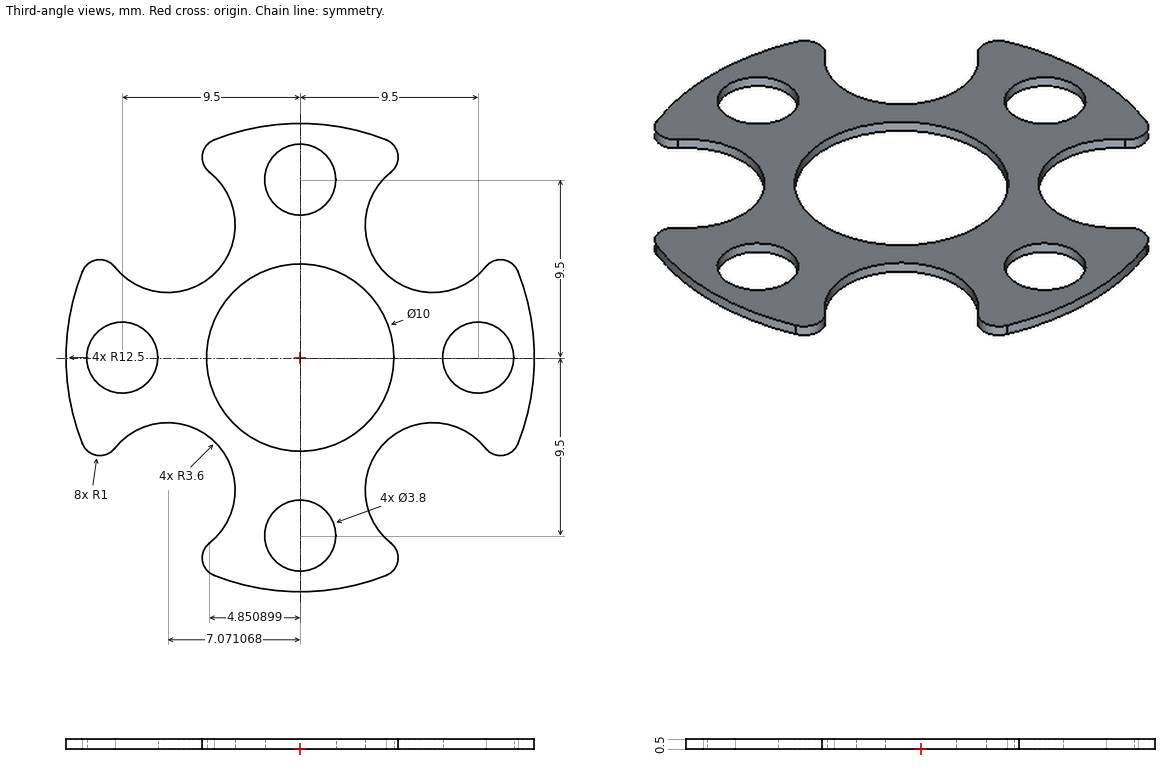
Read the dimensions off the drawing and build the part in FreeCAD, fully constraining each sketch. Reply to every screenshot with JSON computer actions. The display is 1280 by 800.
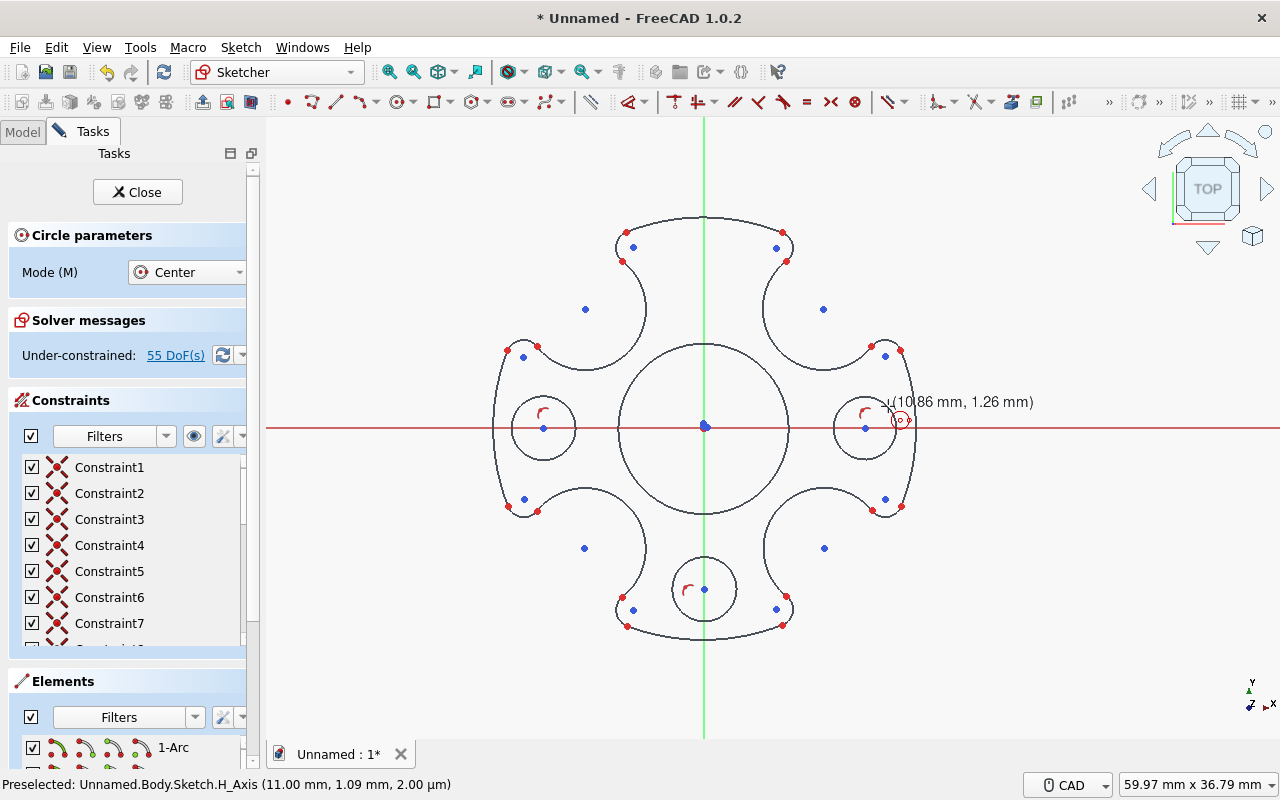
{"action": "left_click", "coordinate": [704, 268]}
{"action": "left_click", "coordinate": [727, 245]}
{"action": "key", "text": "Escape"}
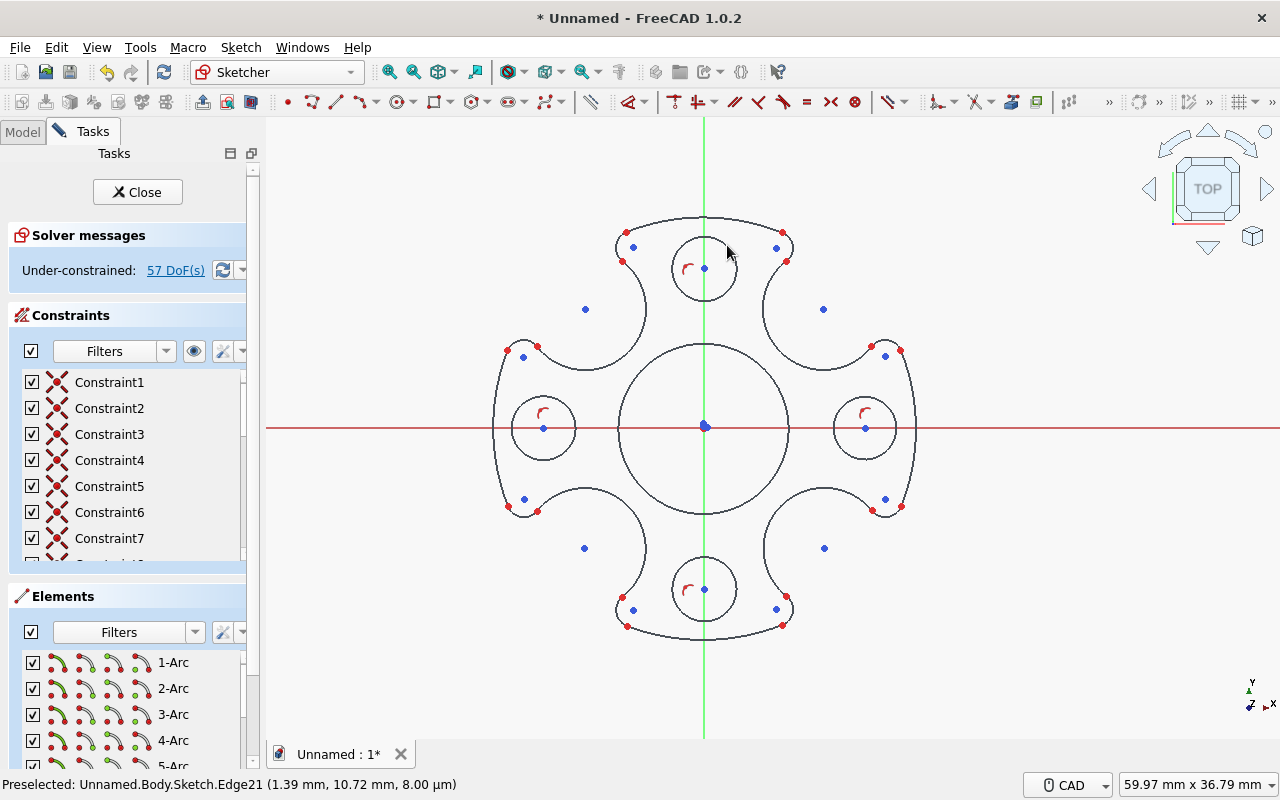
{"action": "left_click", "coordinate": [645, 543]}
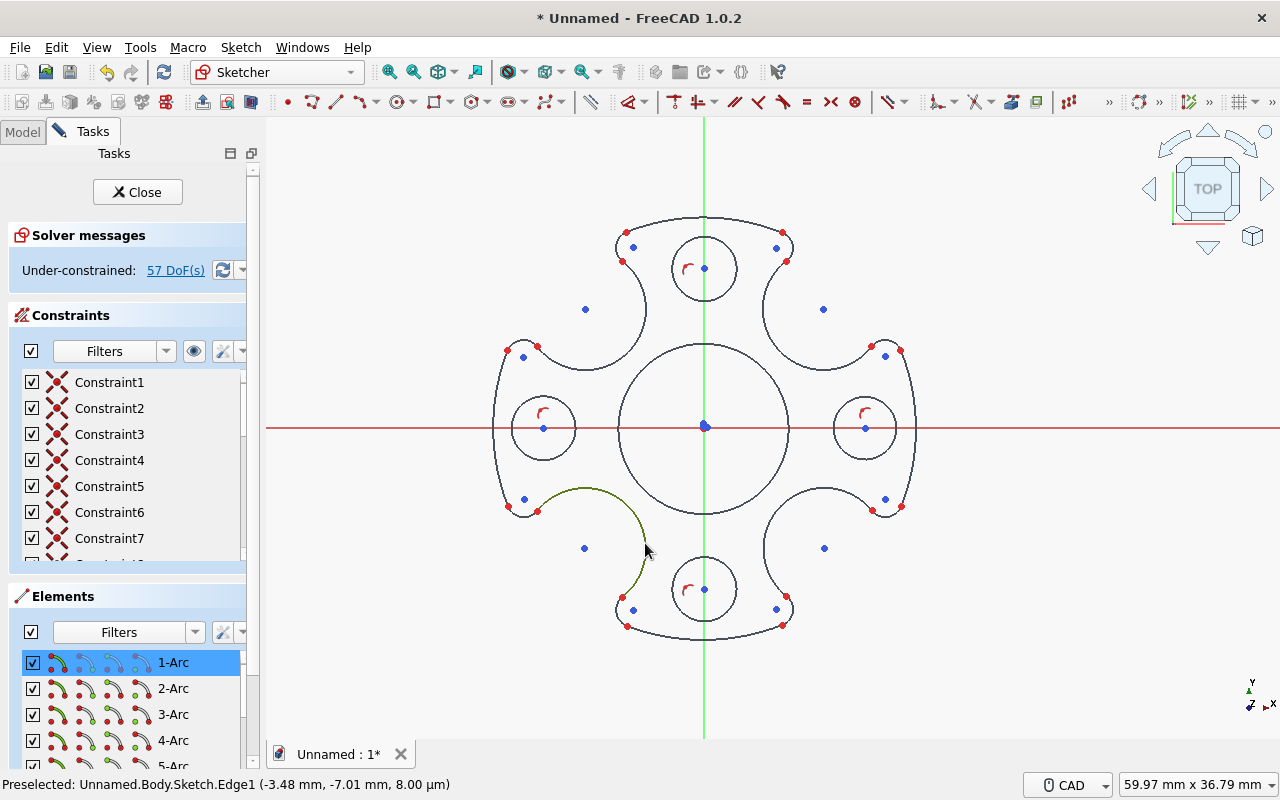
{"action": "scroll", "coordinate": [617, 606], "scroll_direction": "up", "scroll_amount": 2}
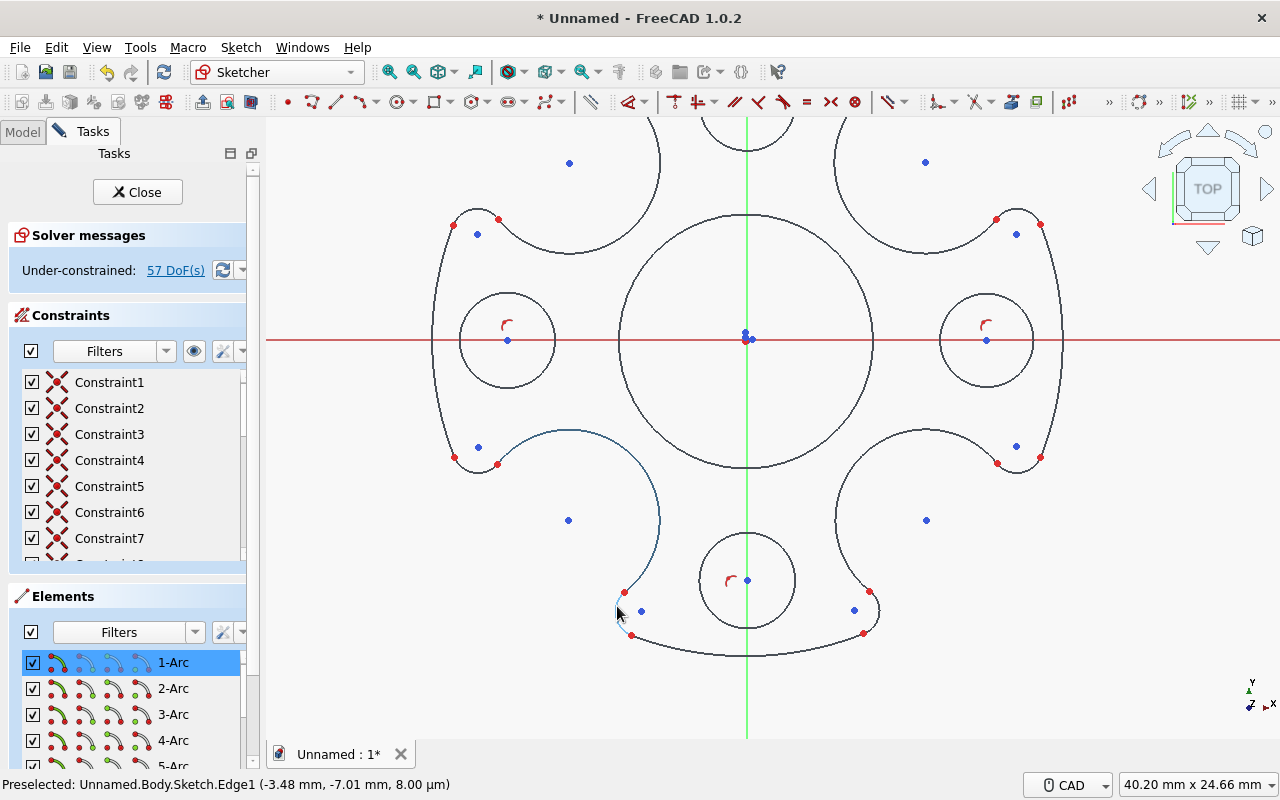
{"action": "left_click", "coordinate": [616, 606]}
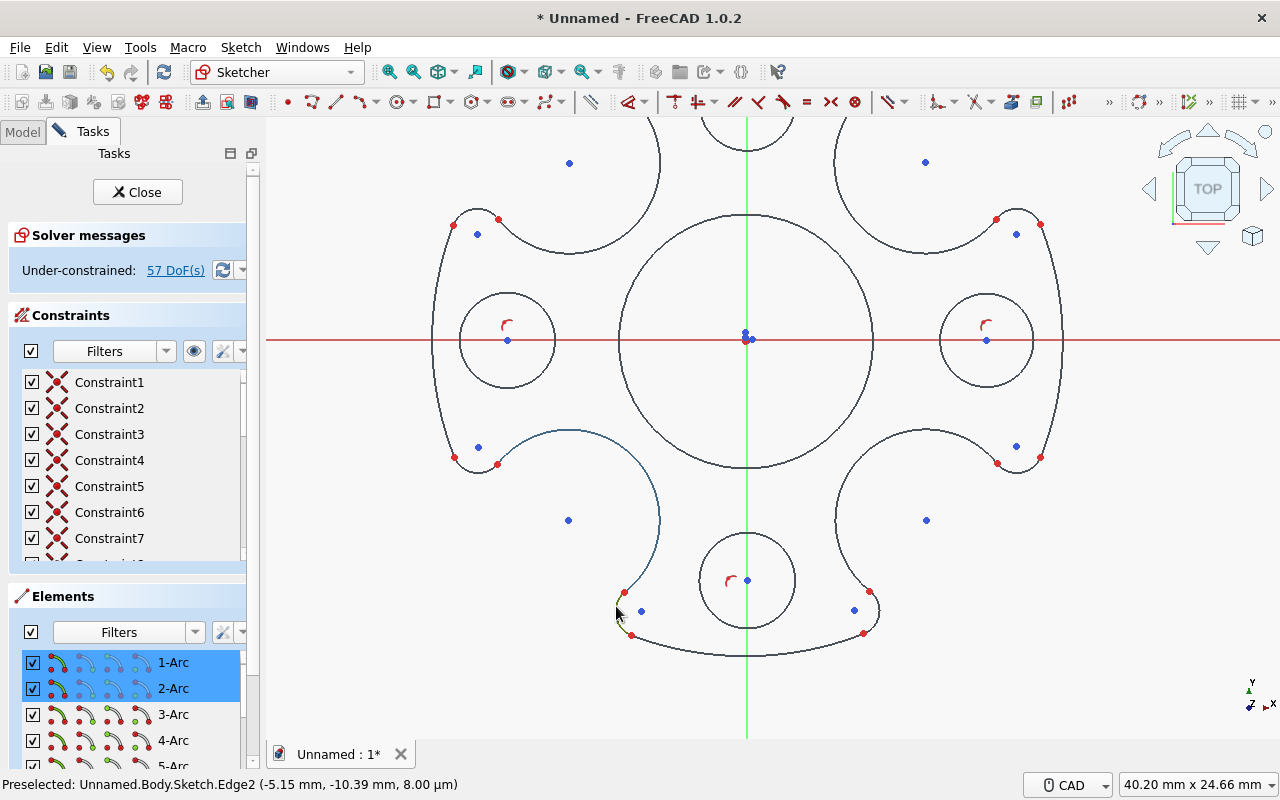
{"action": "left_click", "coordinate": [784, 102]}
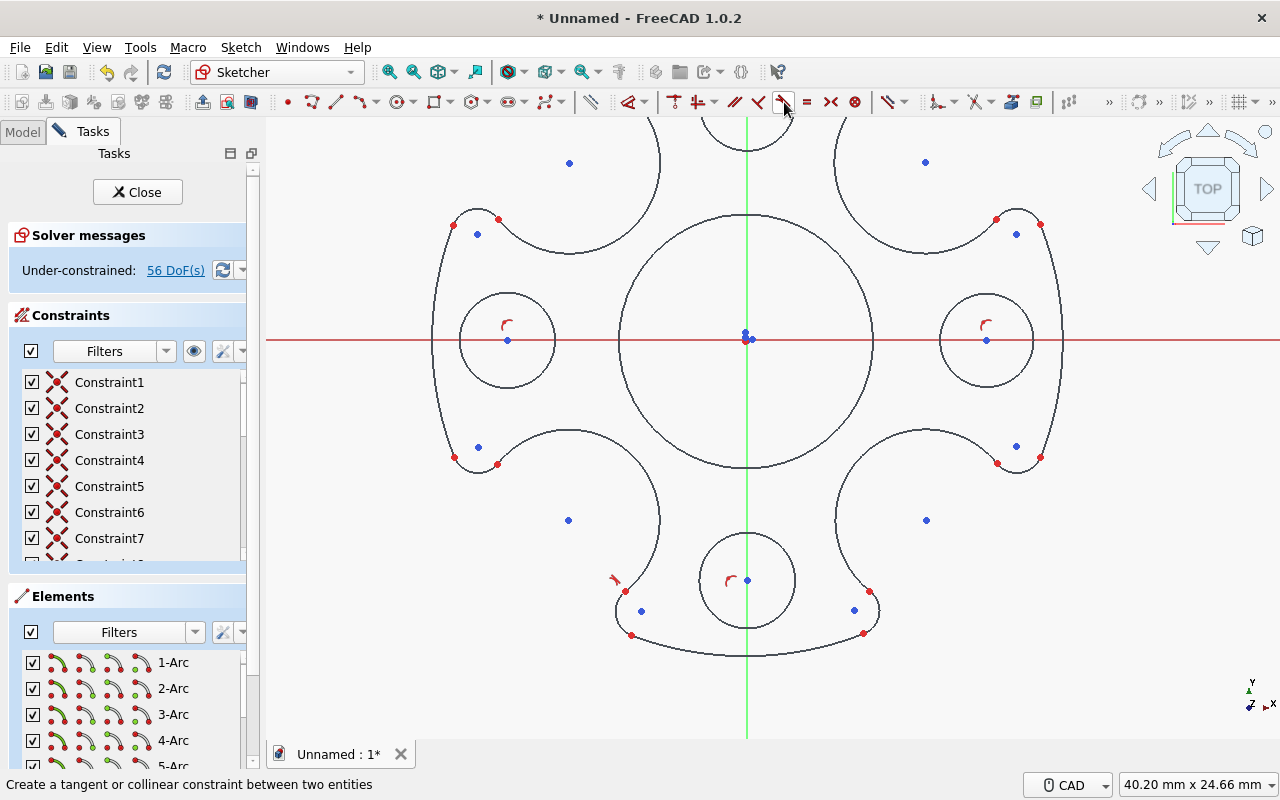
{"action": "left_click", "coordinate": [659, 510]}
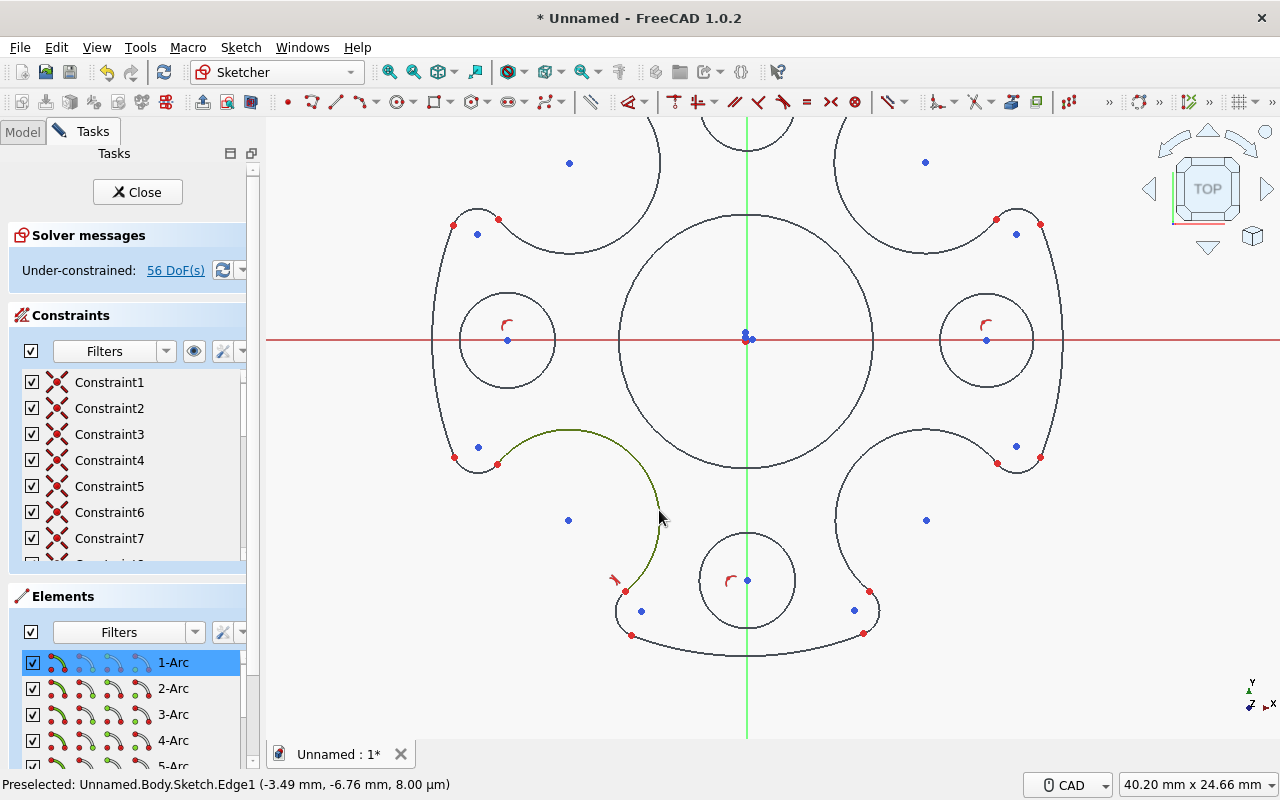
{"action": "left_click", "coordinate": [464, 469]}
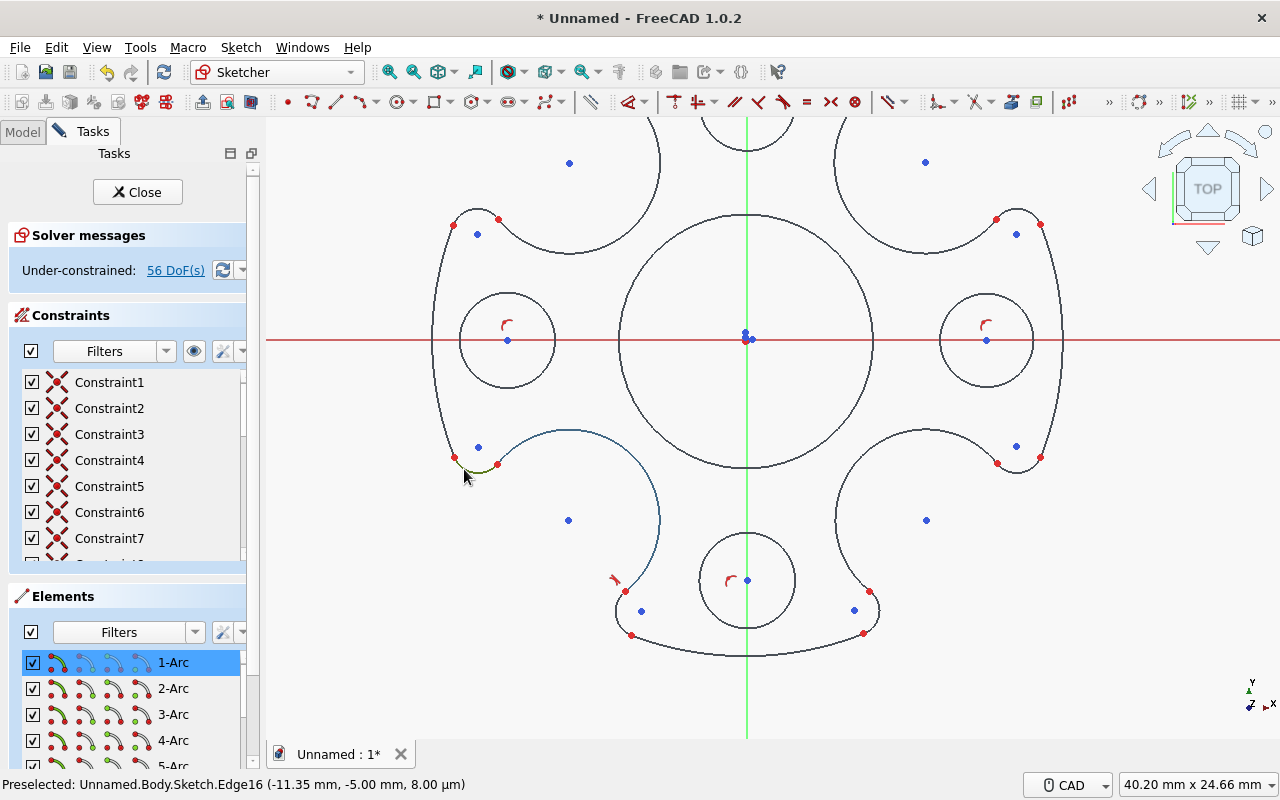
{"action": "key", "text": "t"}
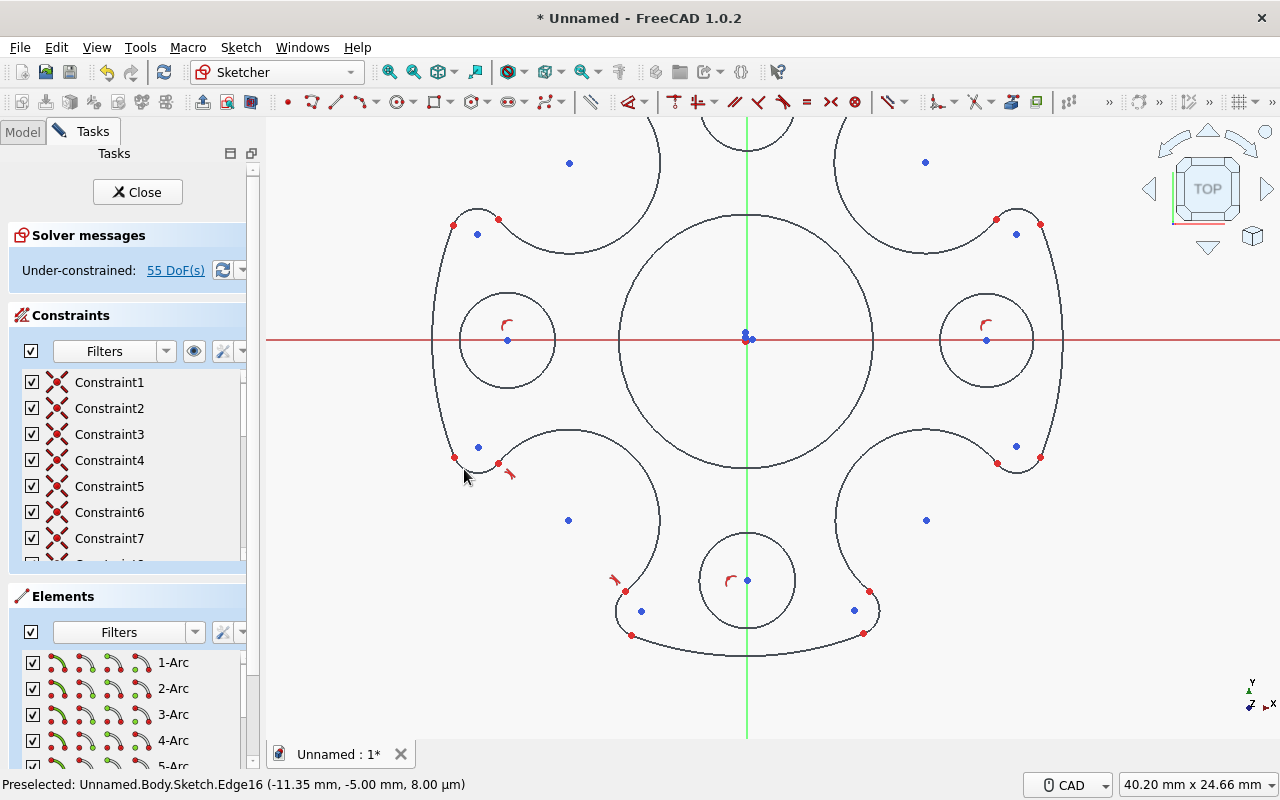
{"action": "left_click", "coordinate": [617, 605]}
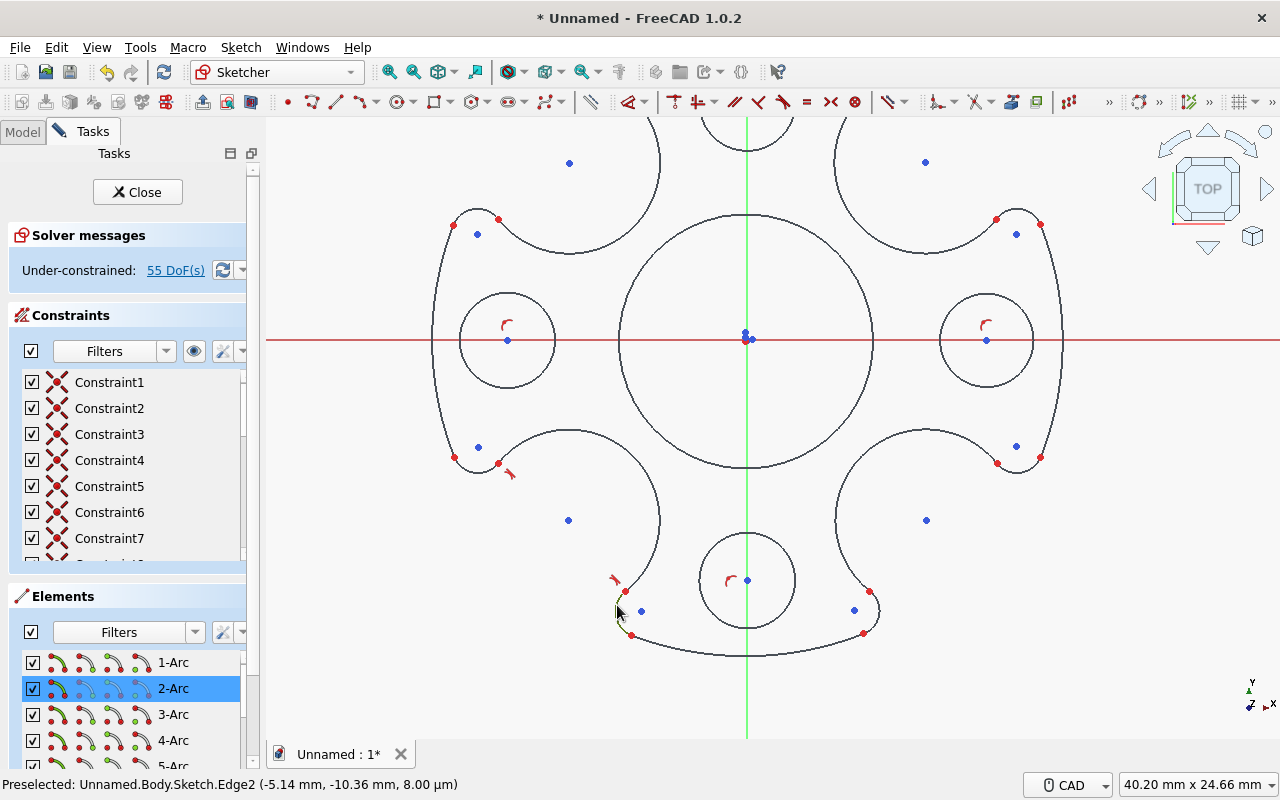
{"action": "left_click", "coordinate": [701, 653]}